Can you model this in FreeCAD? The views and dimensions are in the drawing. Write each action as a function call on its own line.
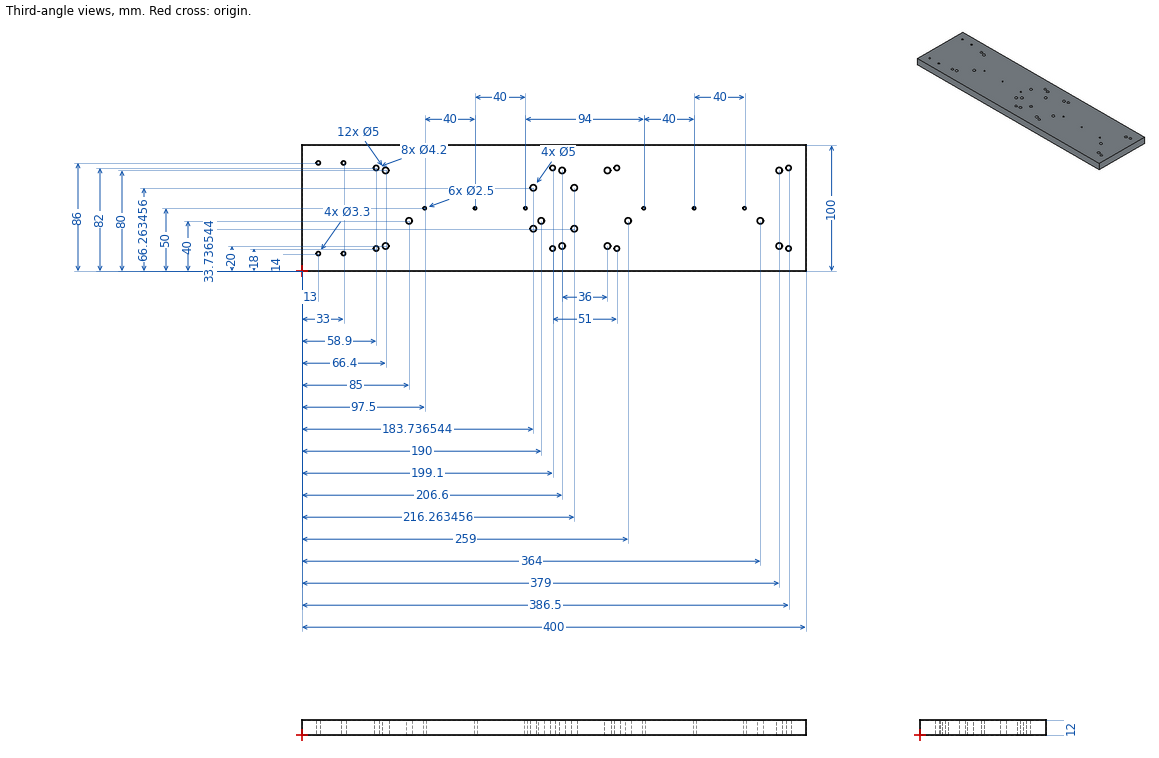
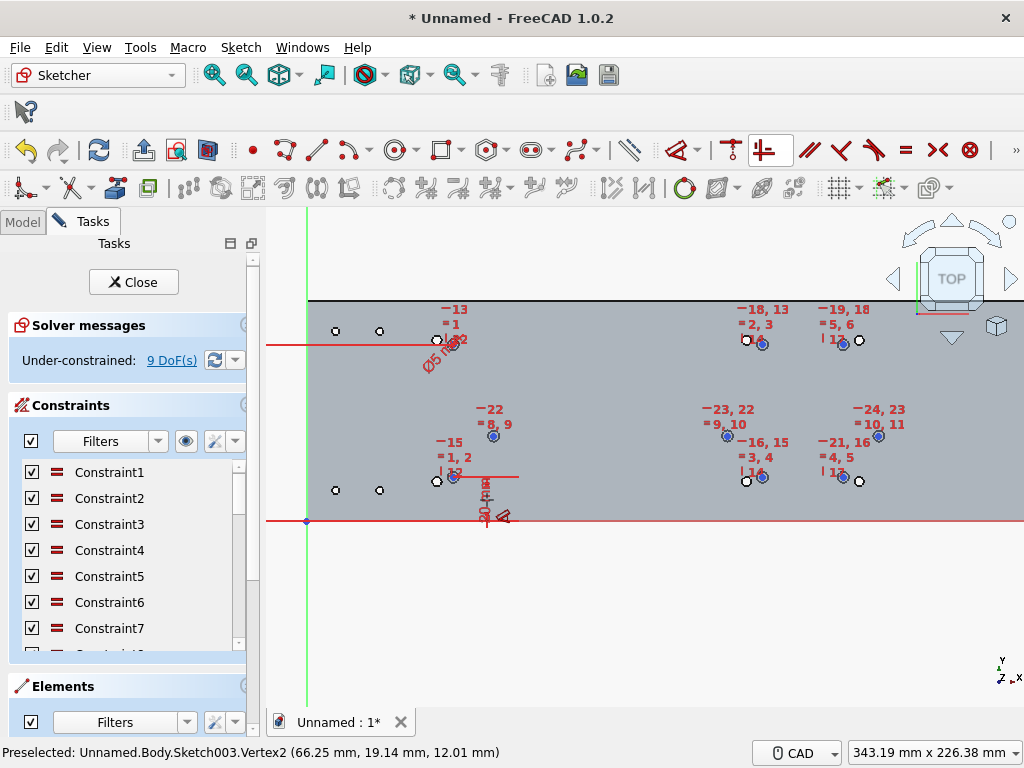
click(494, 436)
click(400, 555)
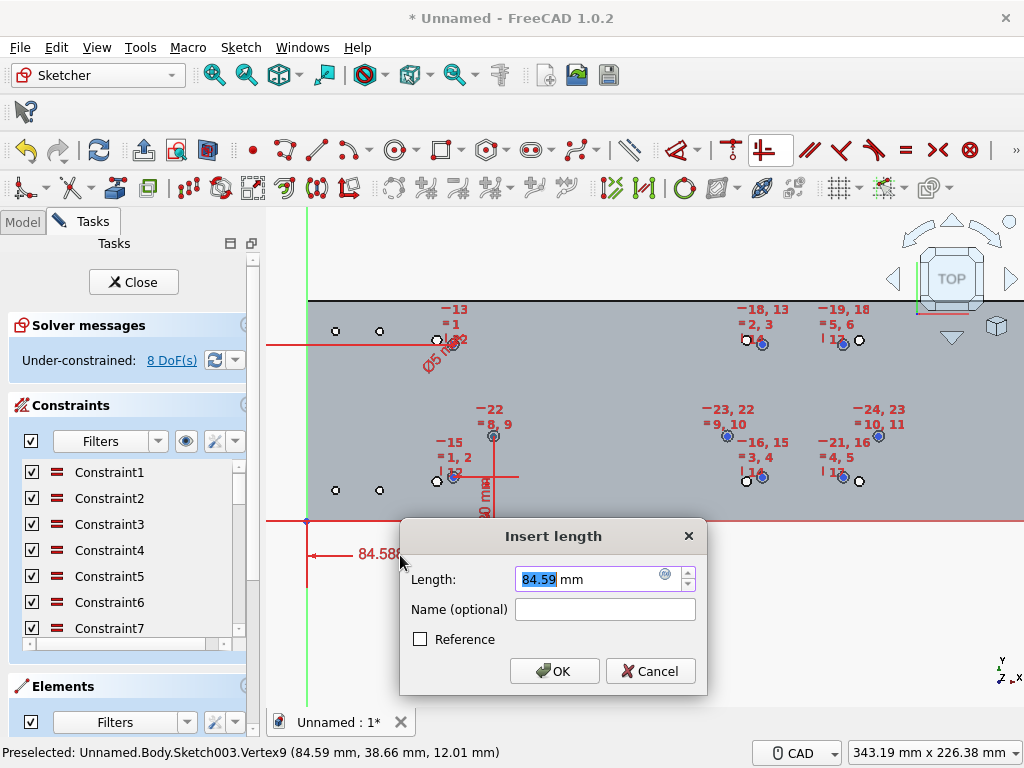
text(85)
key(Return)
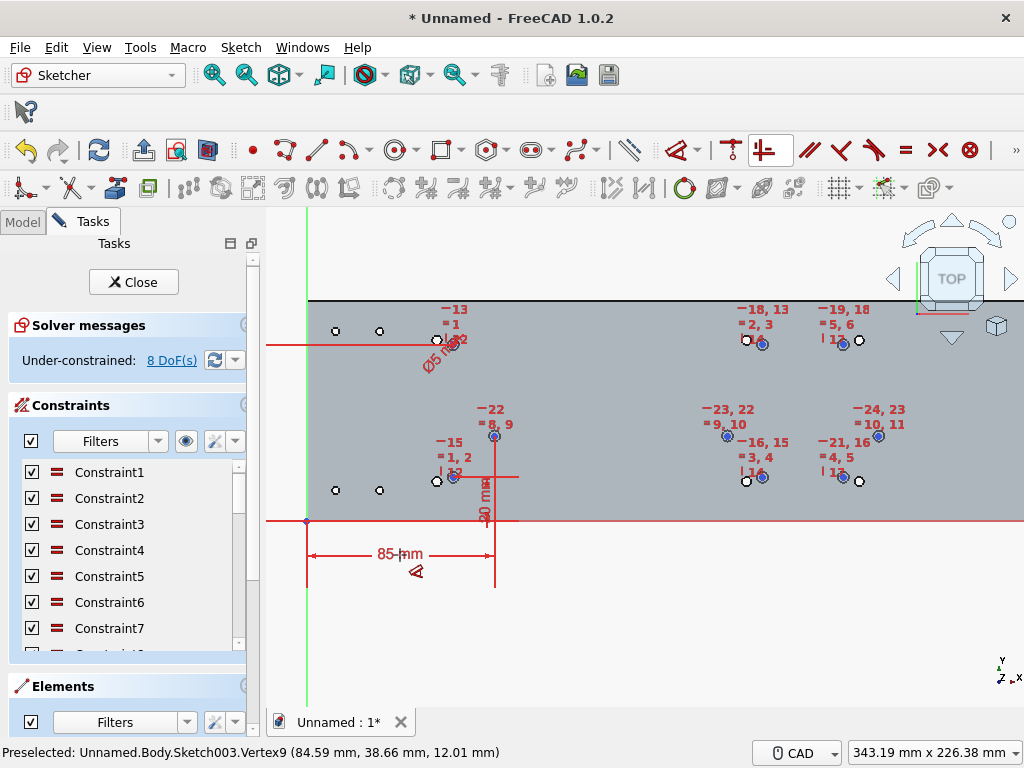
click(495, 436)
click(529, 479)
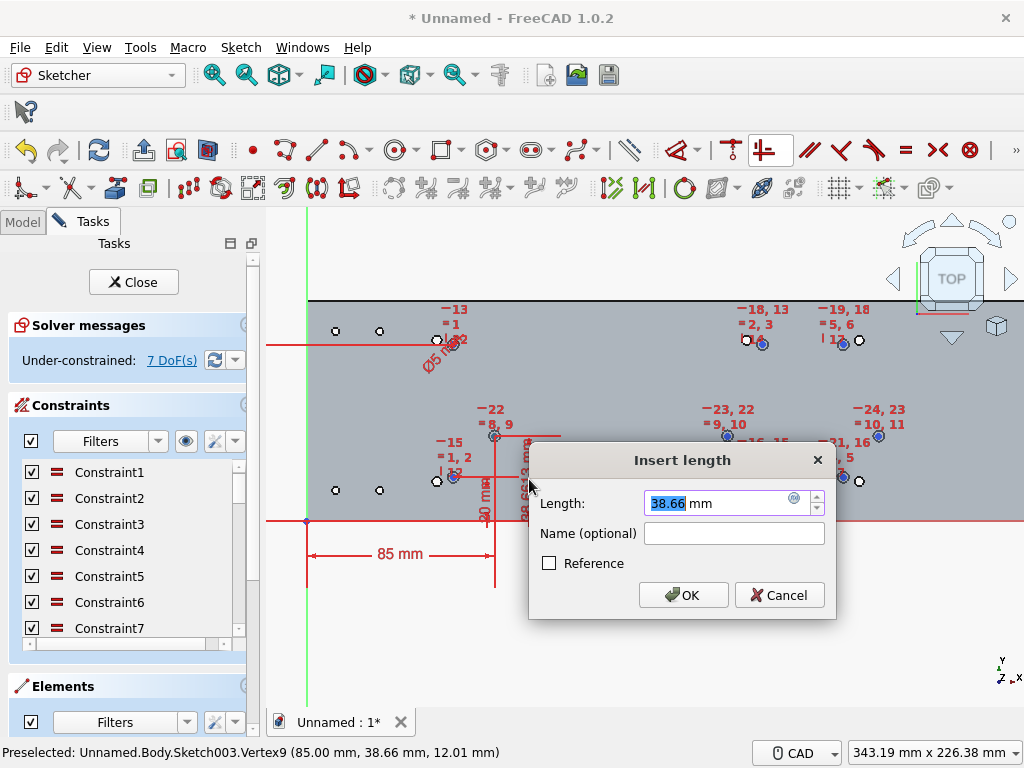
text(40)
key(Return)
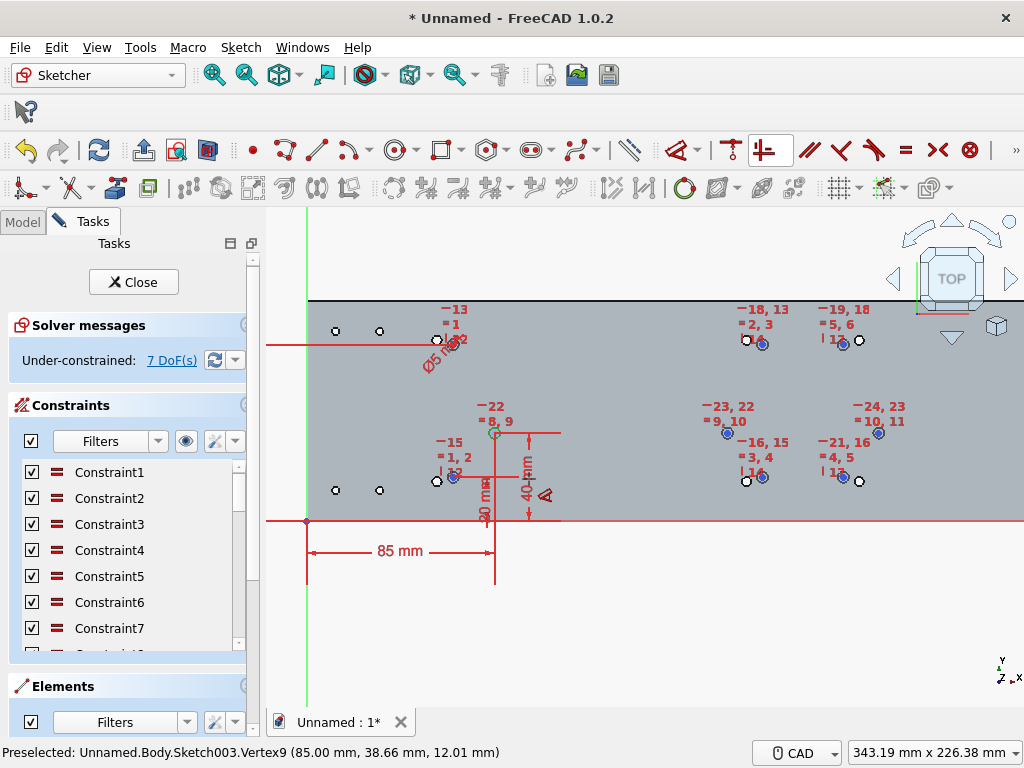
scroll(453, 479, down, 4)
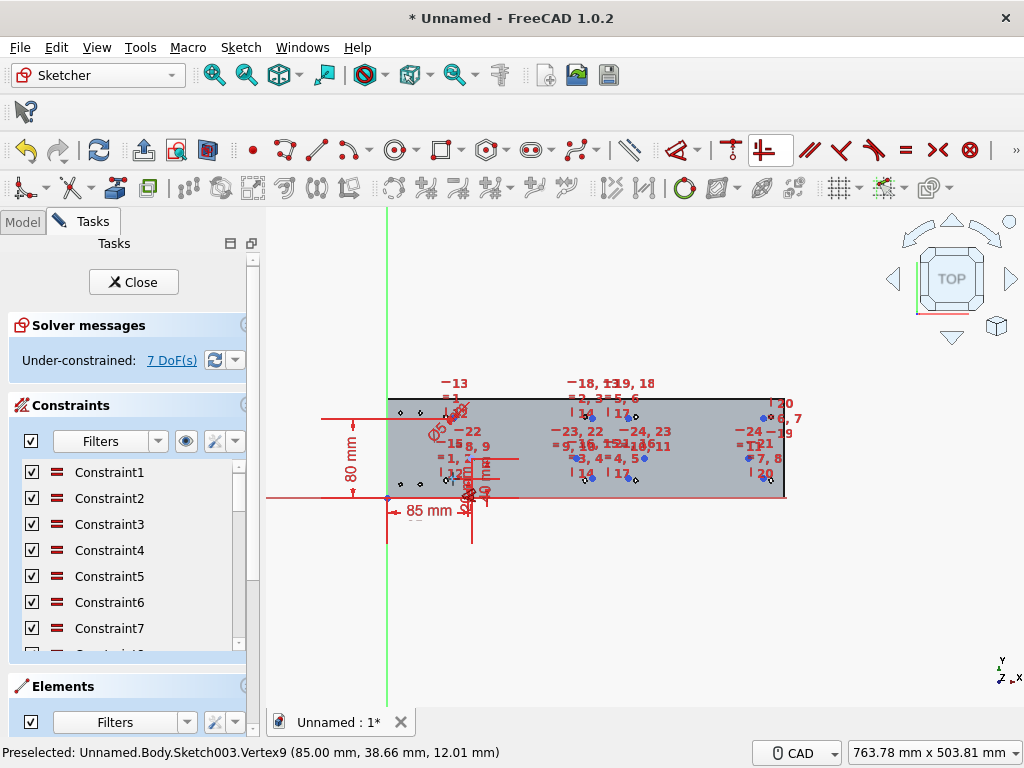
click(763, 419)
click(575, 532)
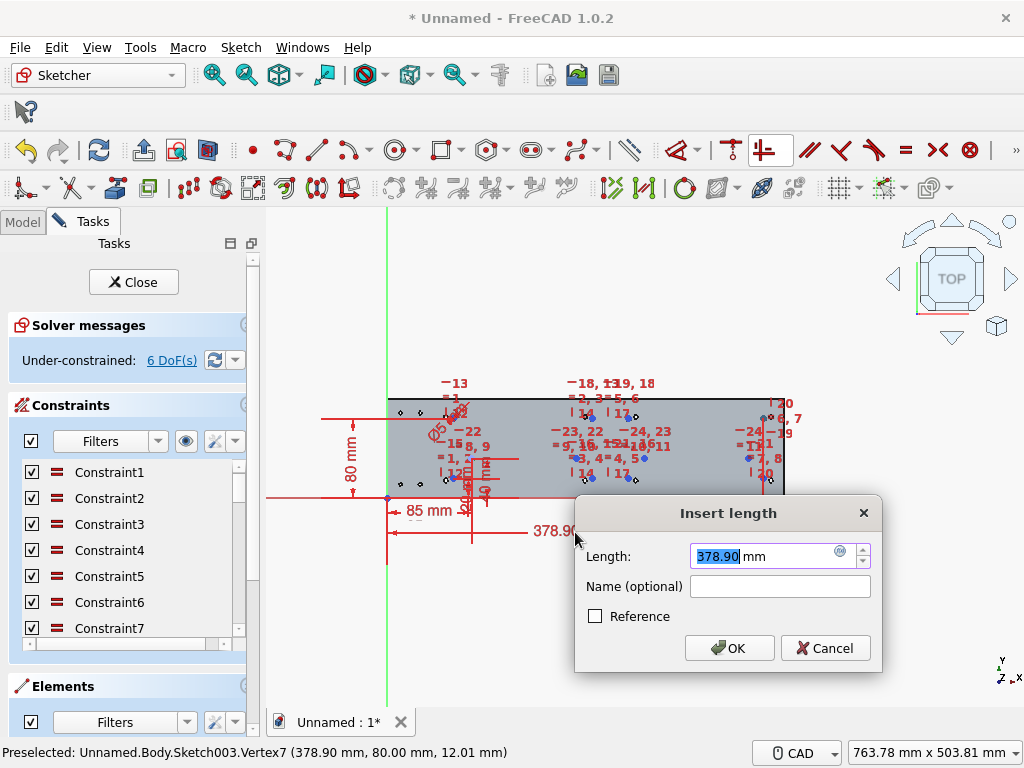
text(379)
key(Return)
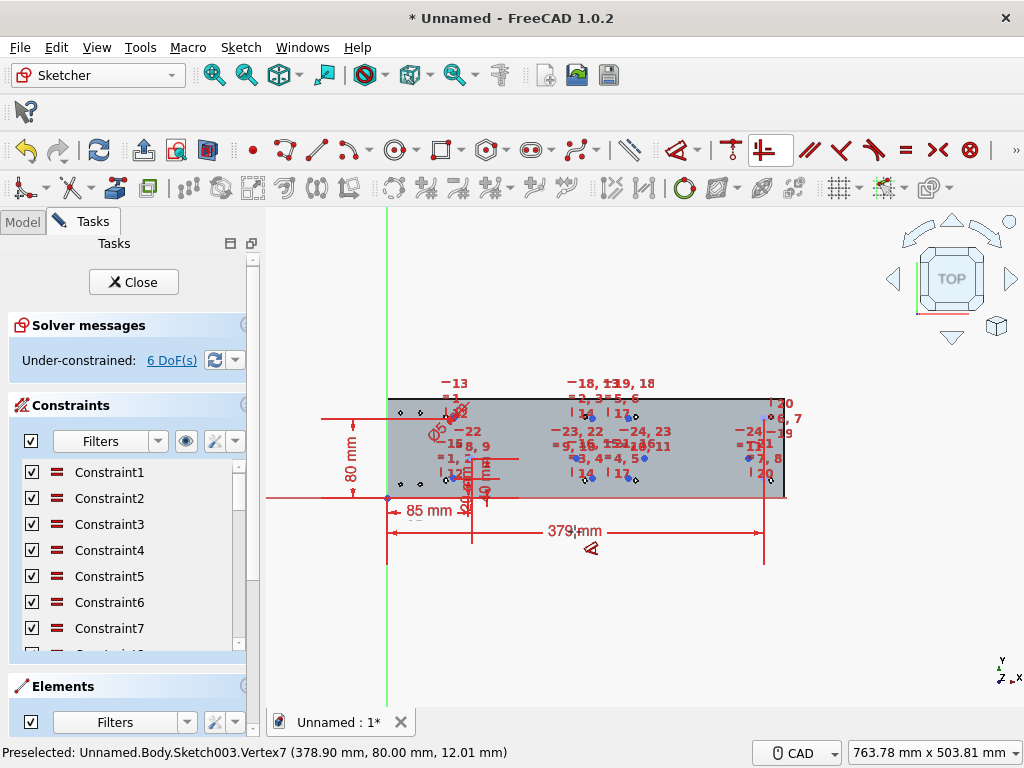
click(576, 459)
click(525, 425)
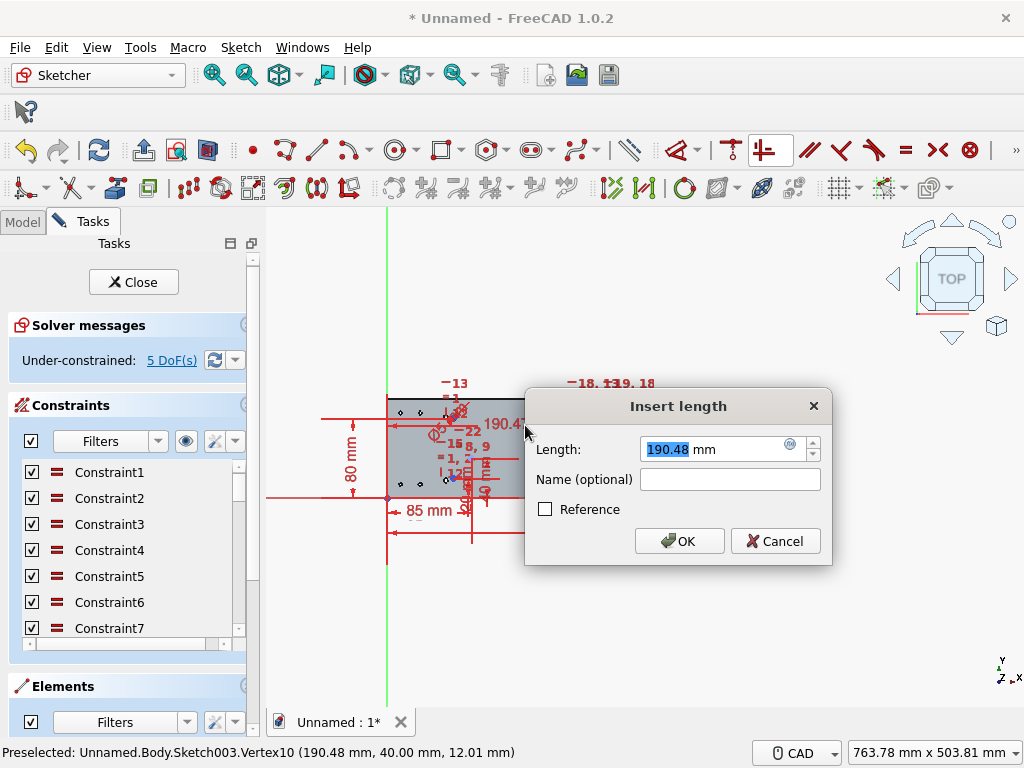
text(190)
key(Return)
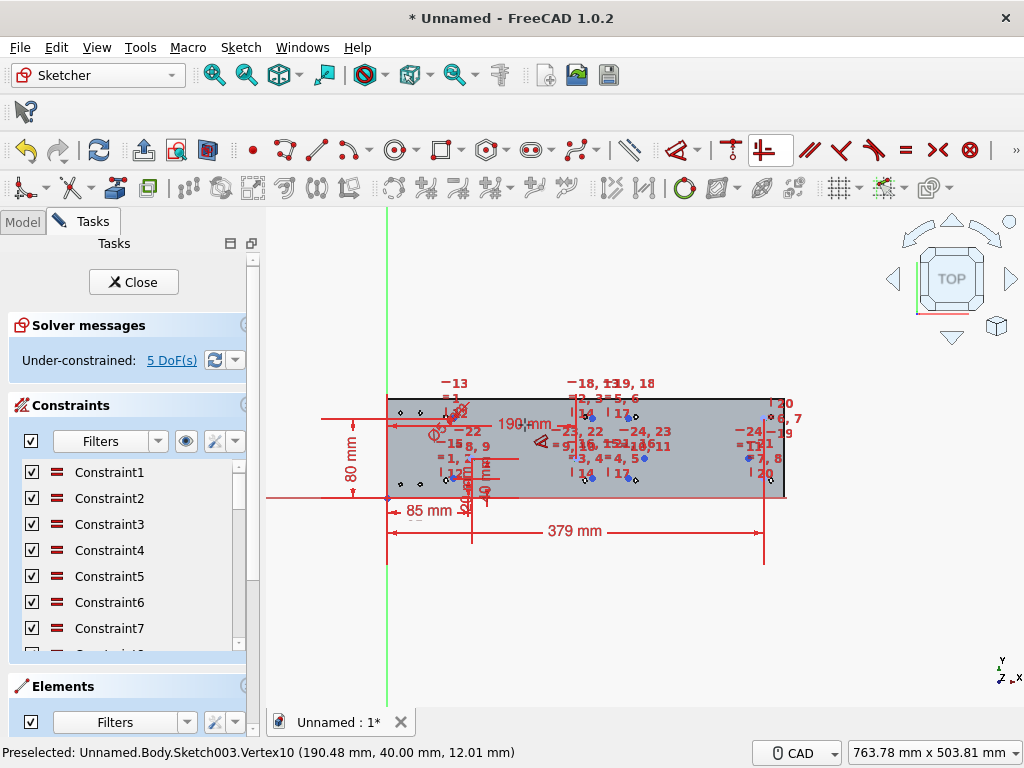
click(644, 459)
click(516, 556)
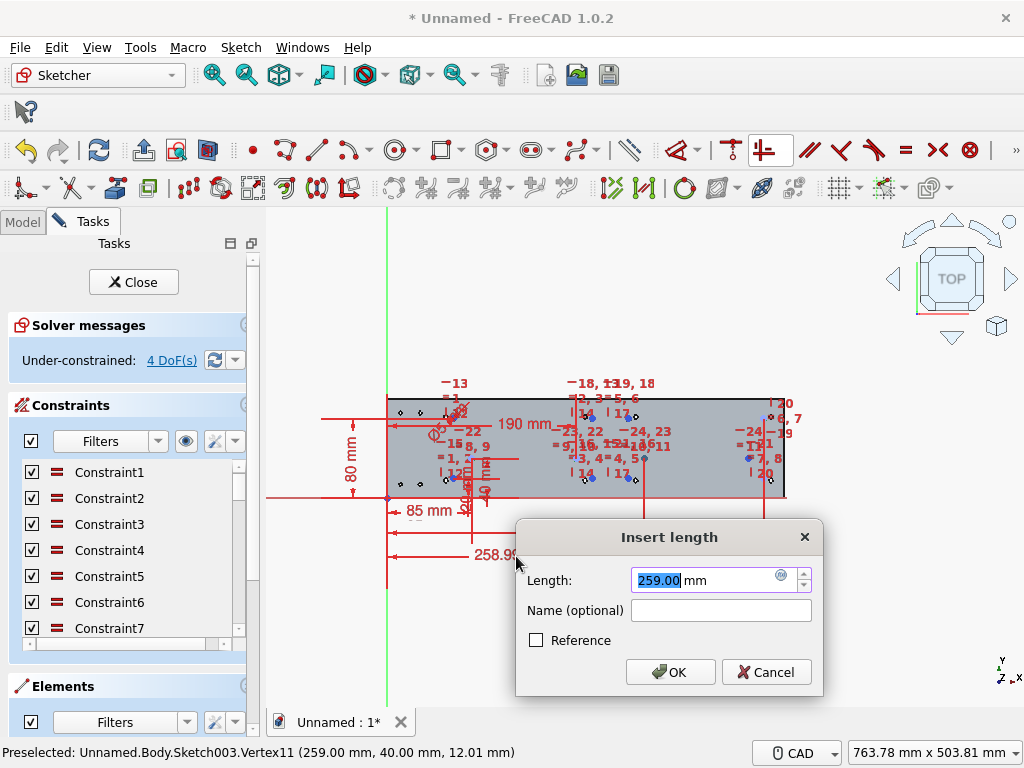
text(259)
key(Return)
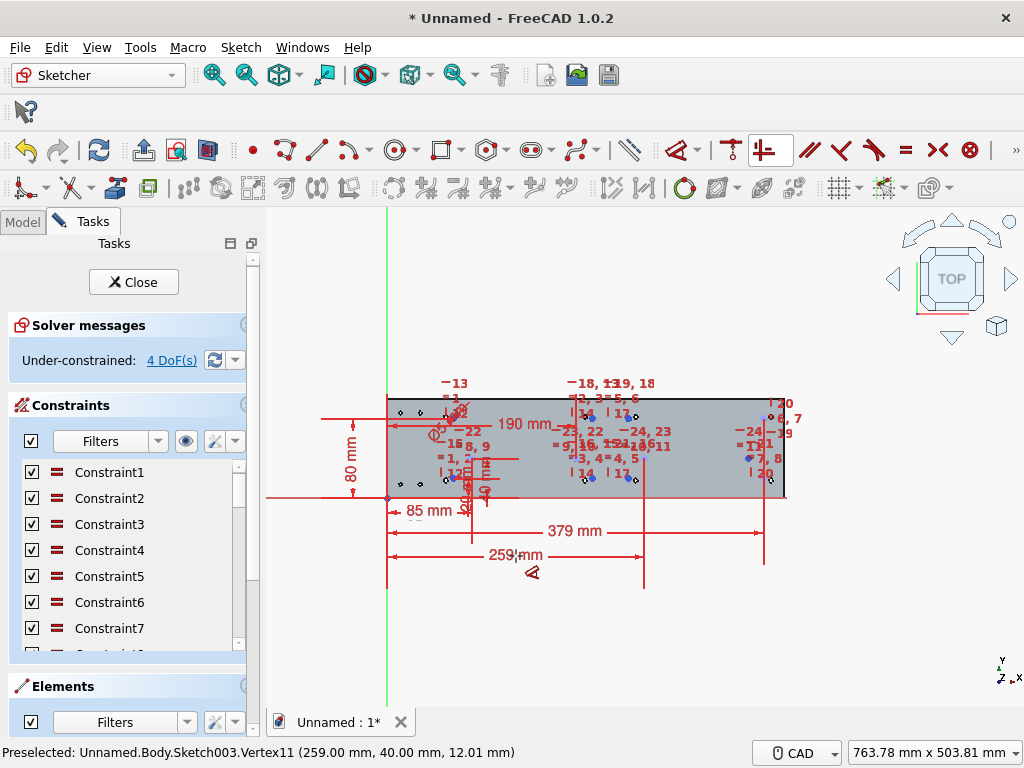
click(748, 459)
click(651, 532)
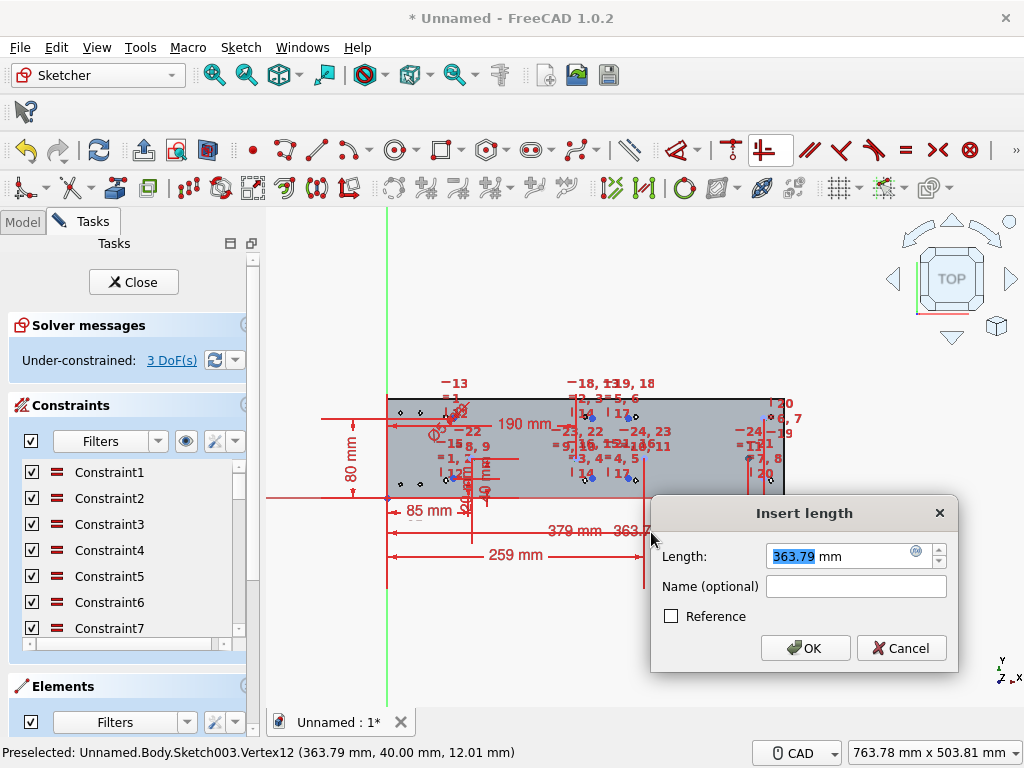
text(364)
key(Return)